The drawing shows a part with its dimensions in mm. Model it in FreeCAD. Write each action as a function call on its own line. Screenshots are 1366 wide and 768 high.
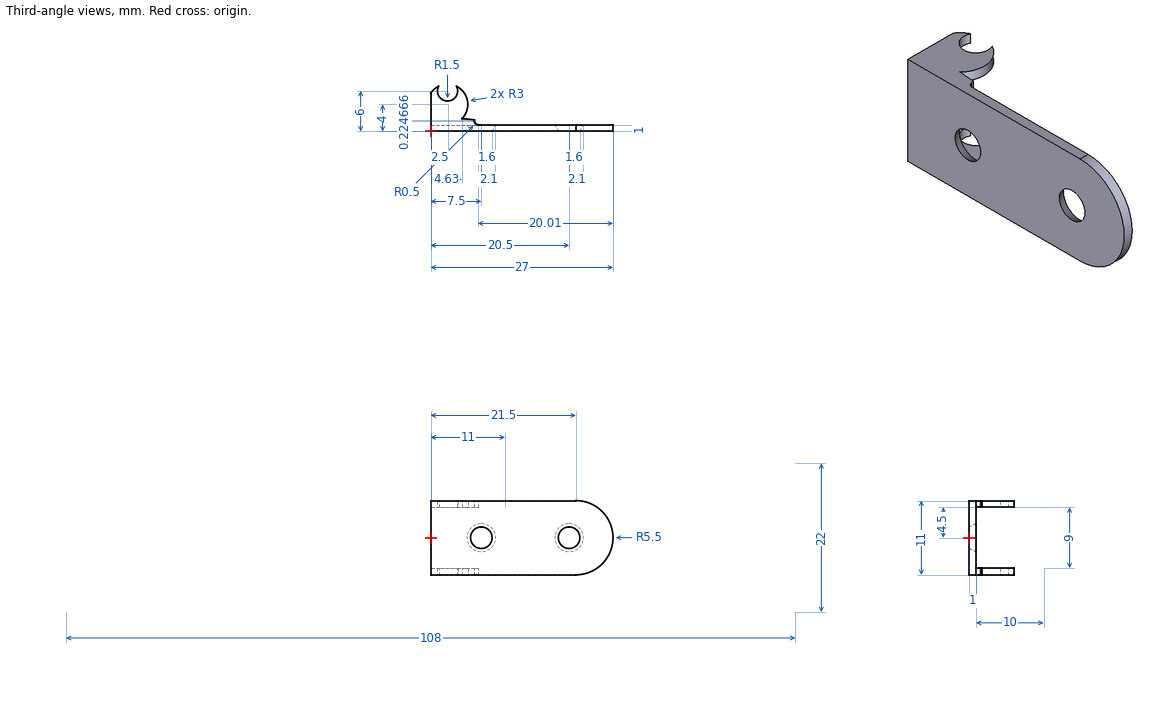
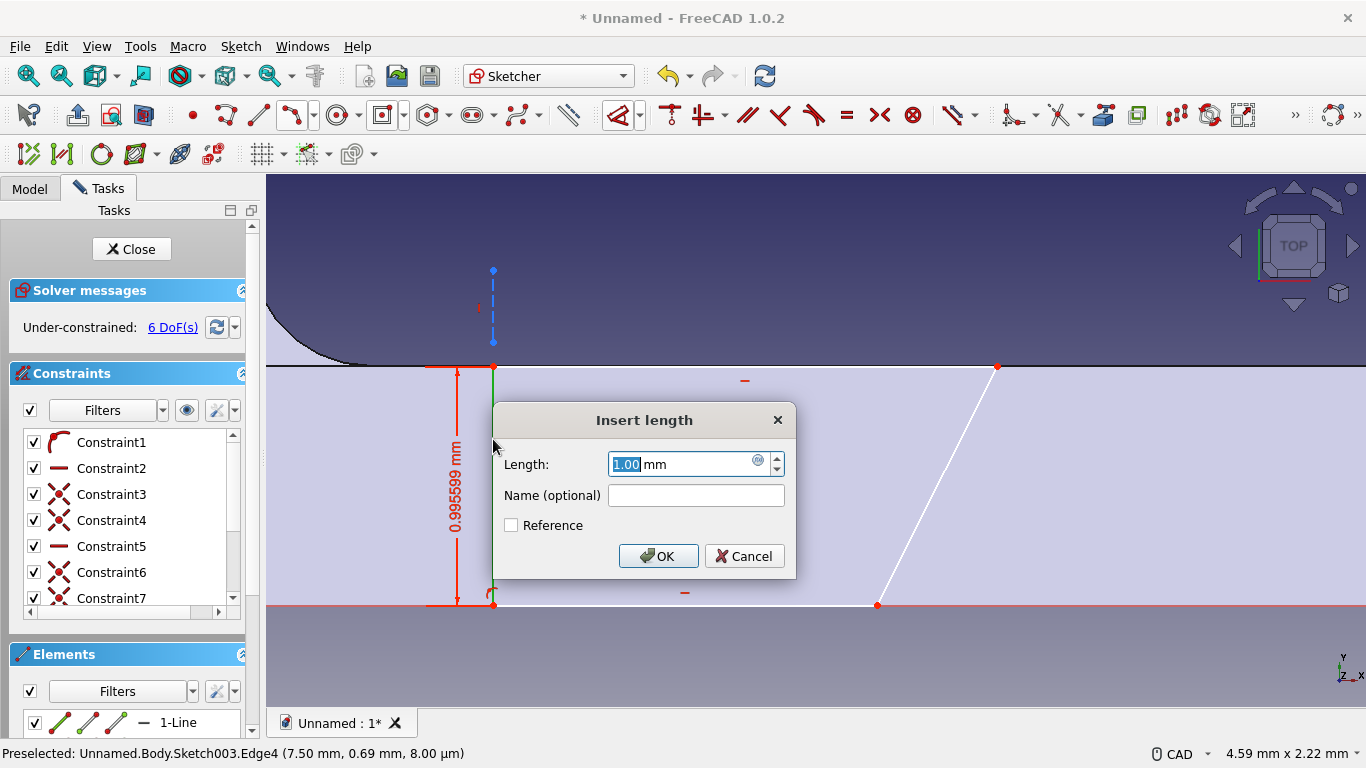
text(1)
key(Return)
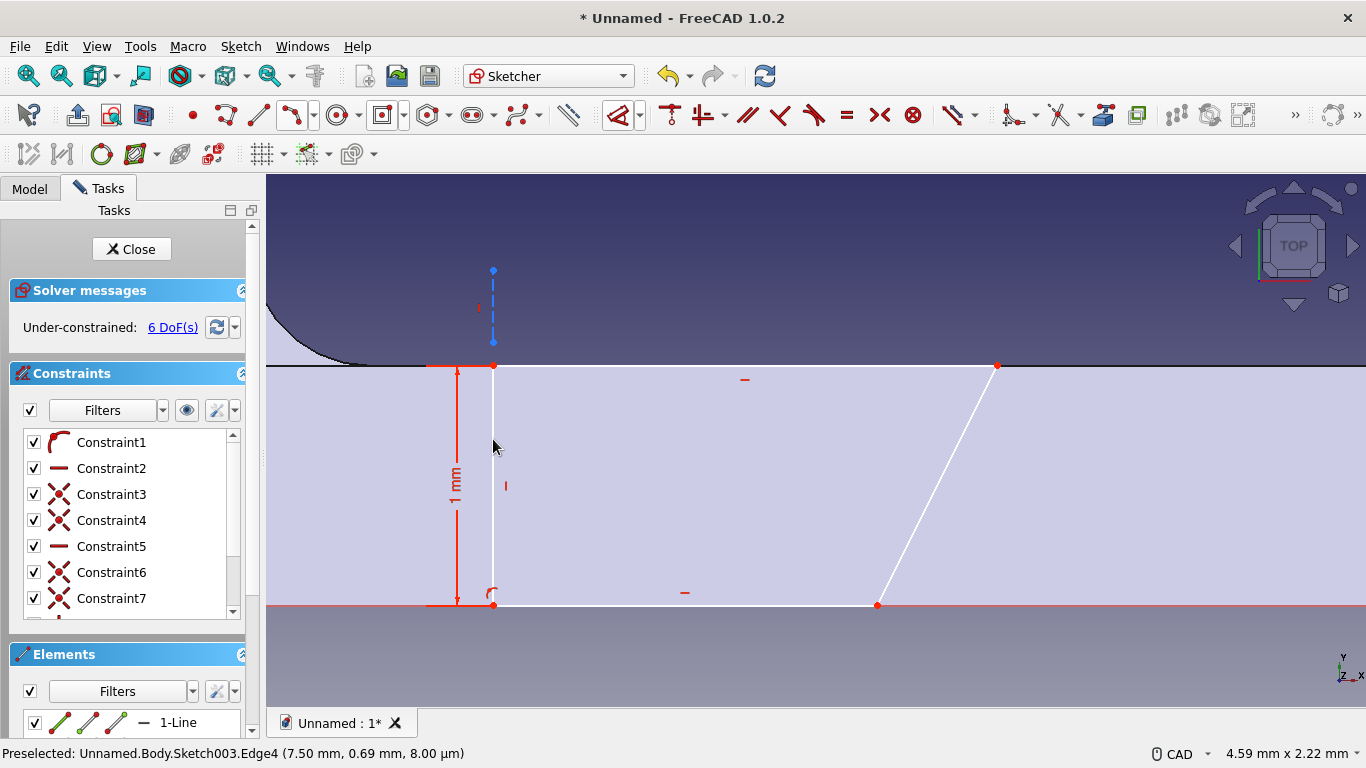
click(608, 606)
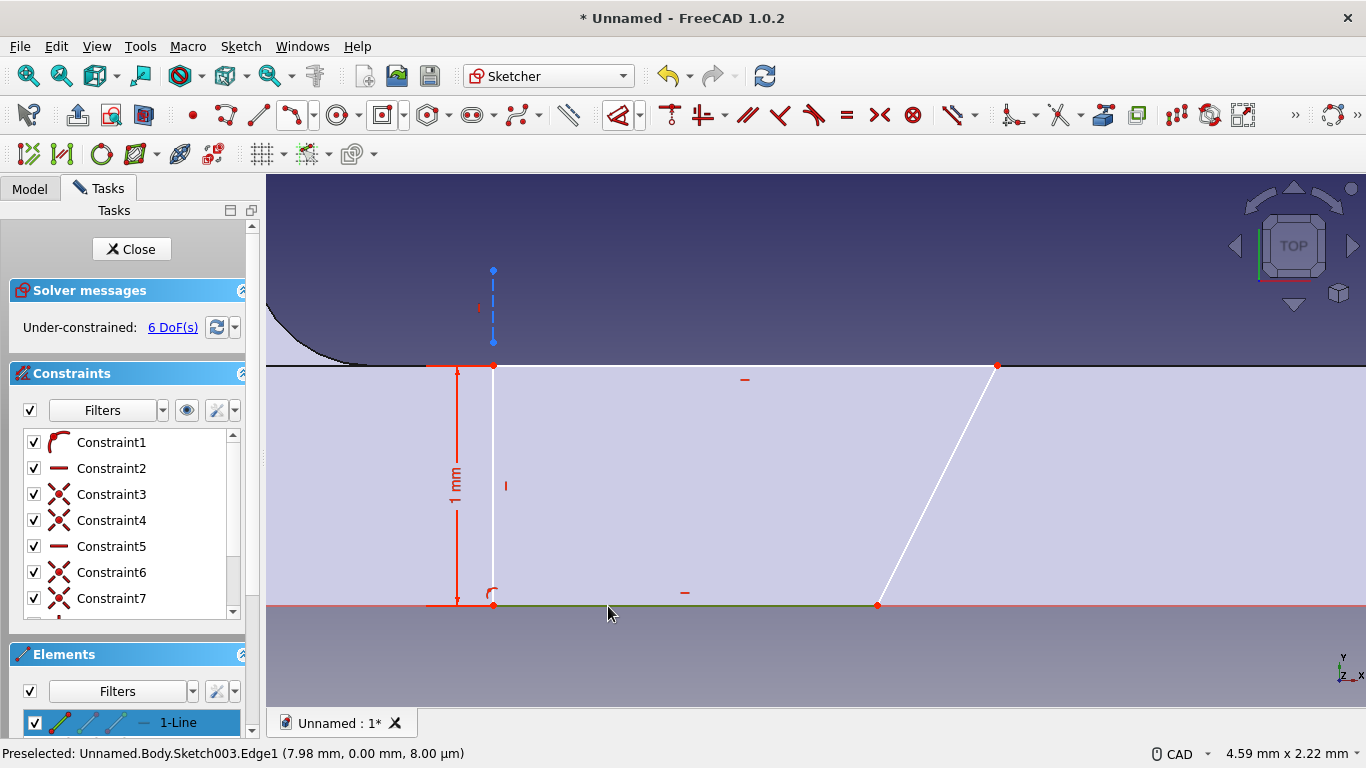
key(l)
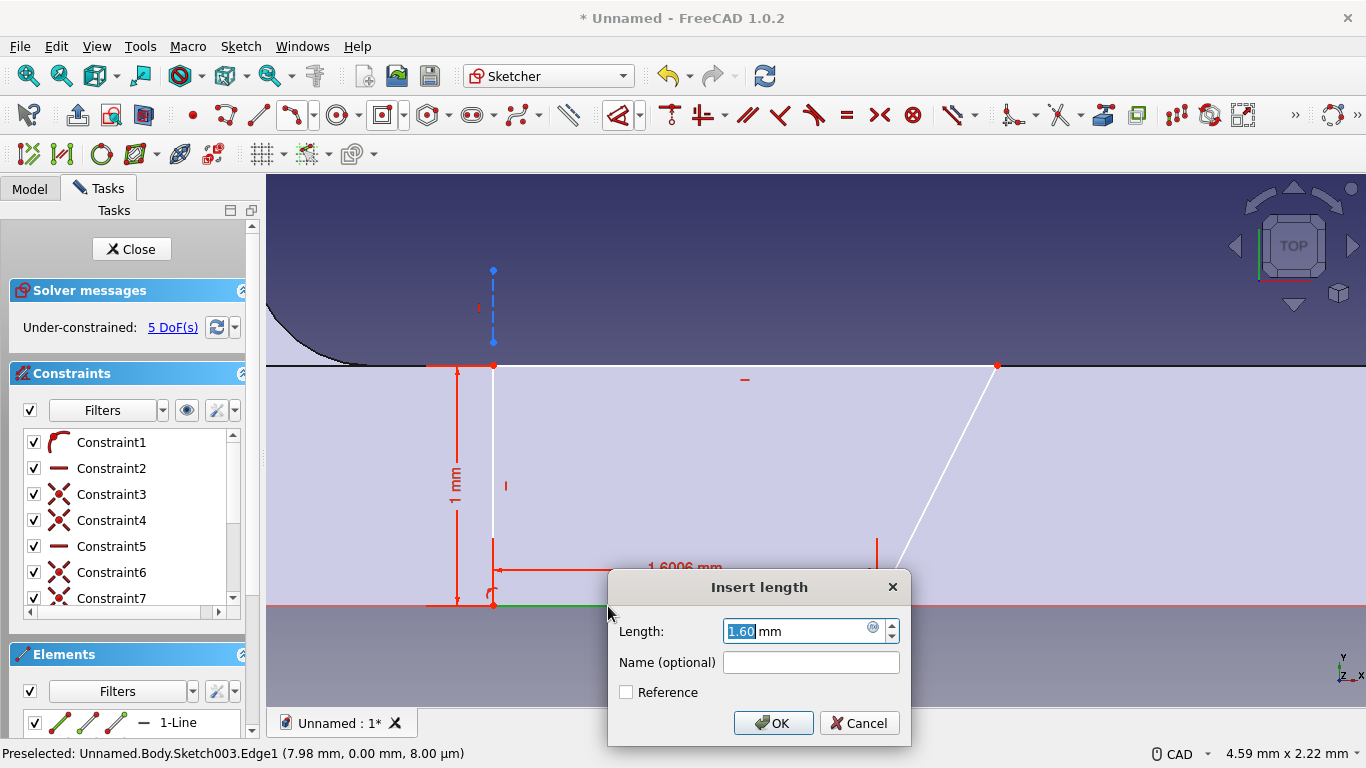
text(1.6)
key(Return)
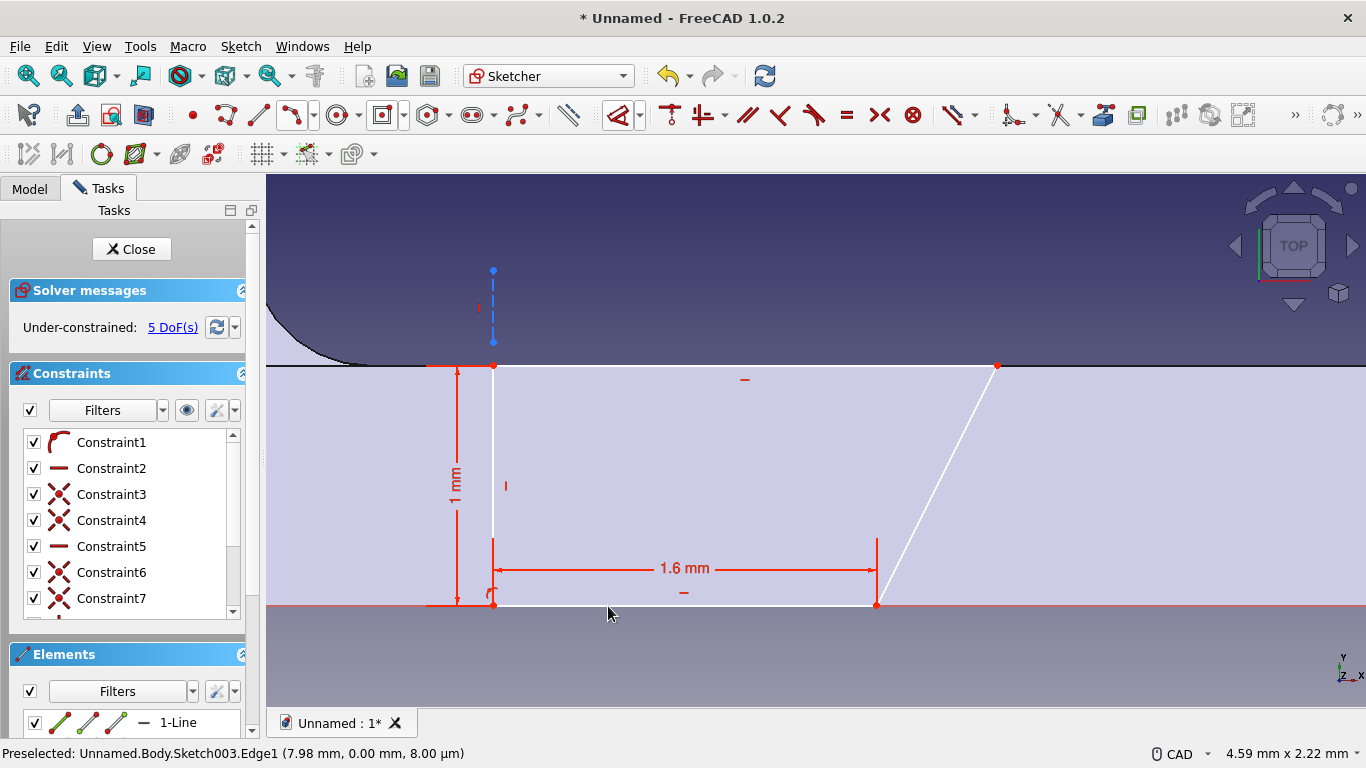
click(846, 366)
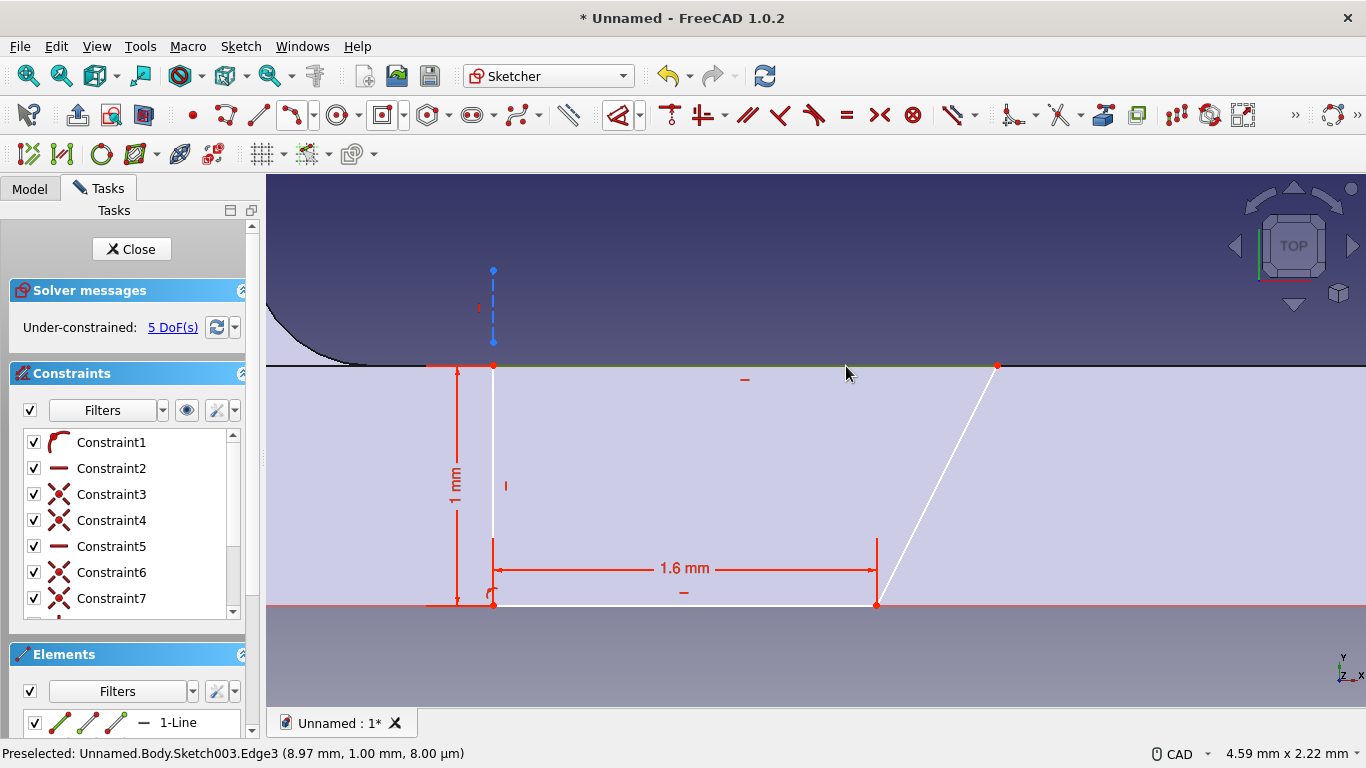
key(l)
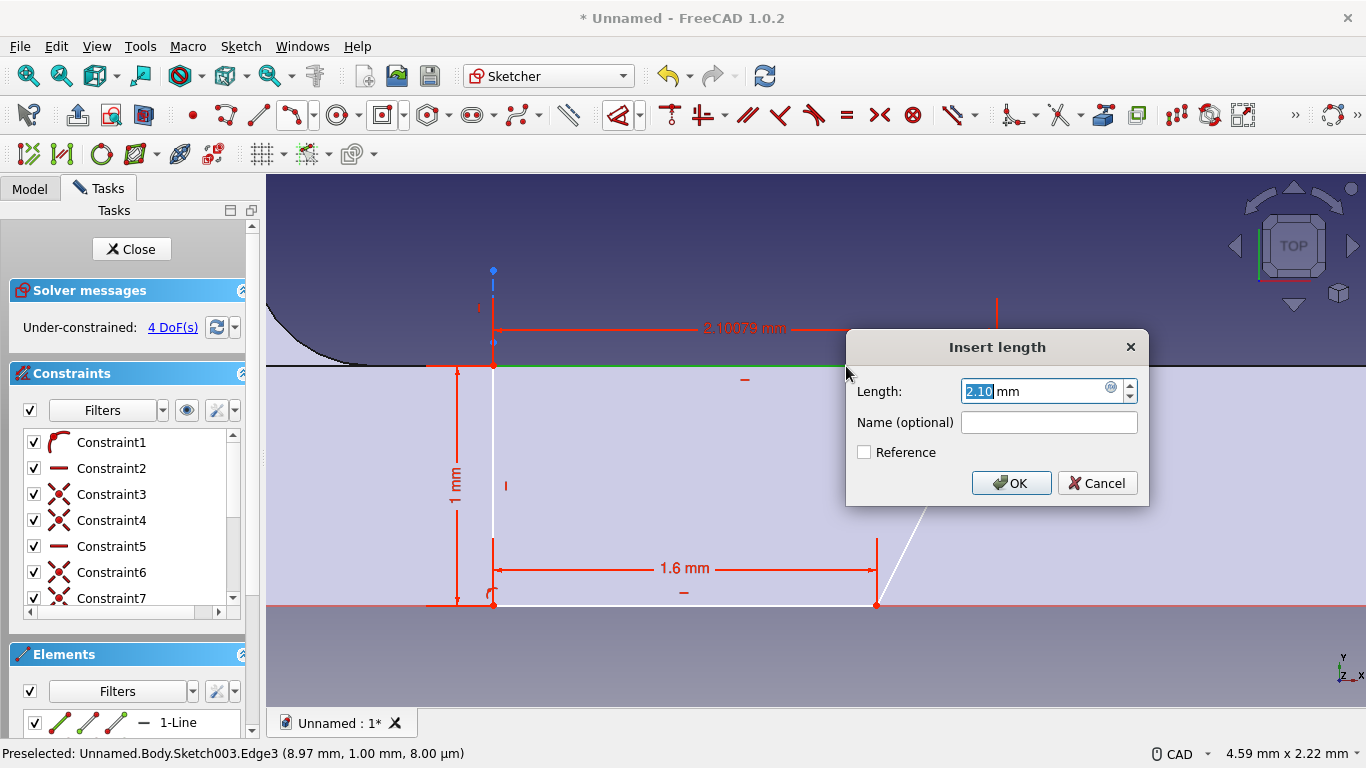
text(2.1)
key(Return)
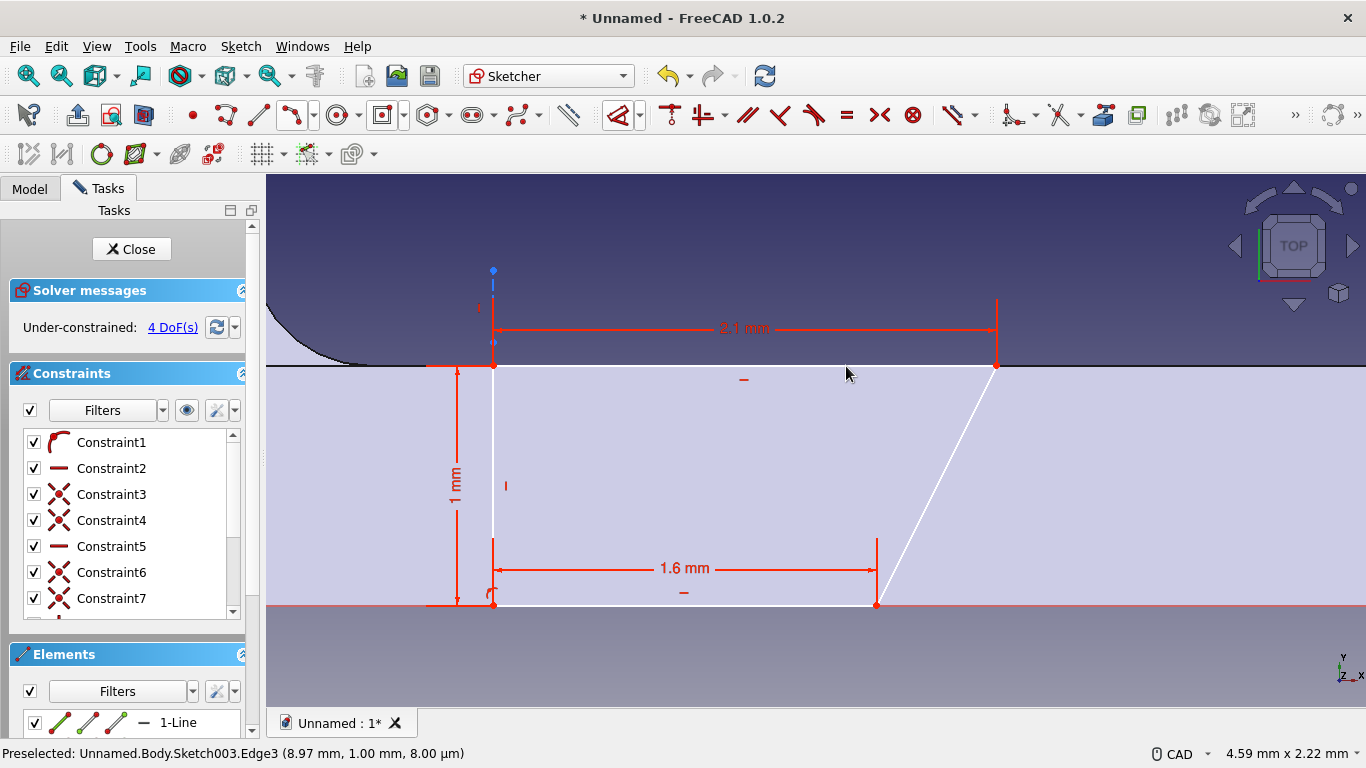
click(493, 606)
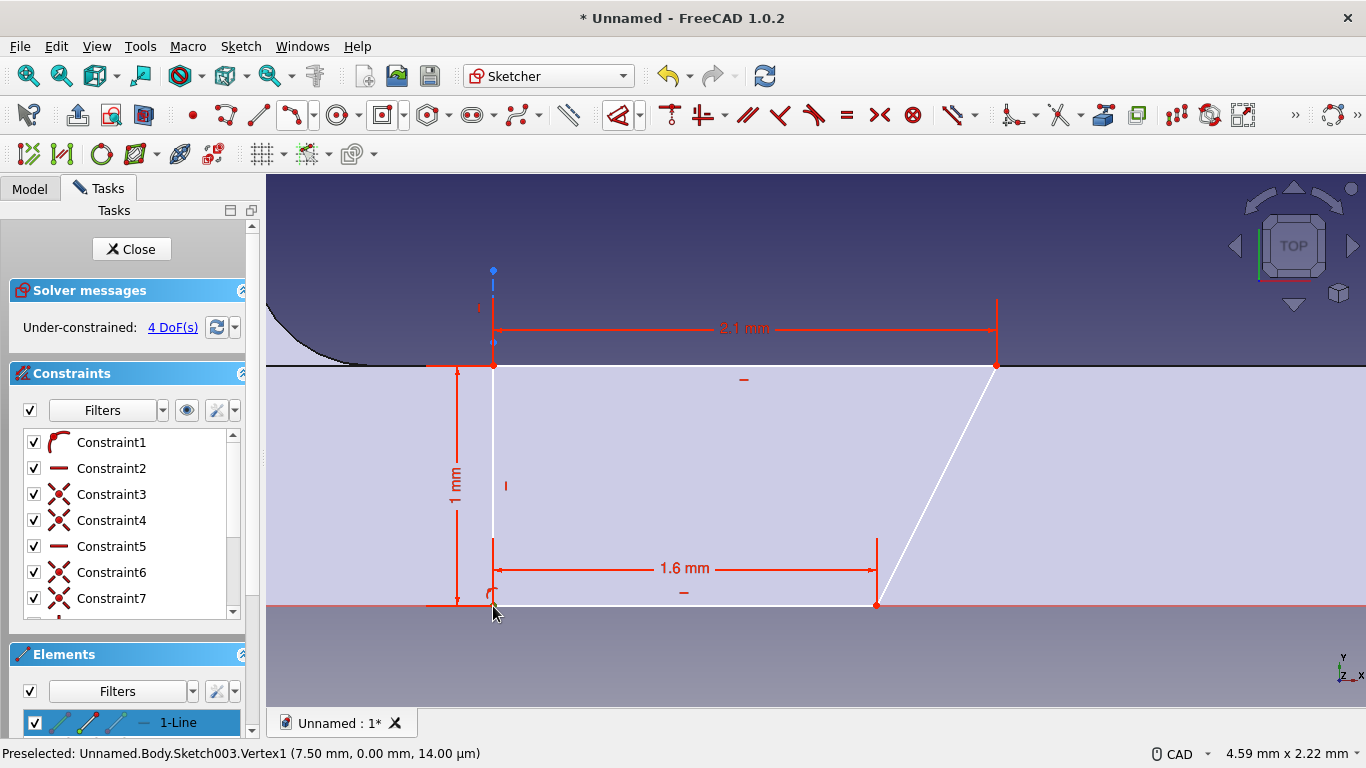
key(l)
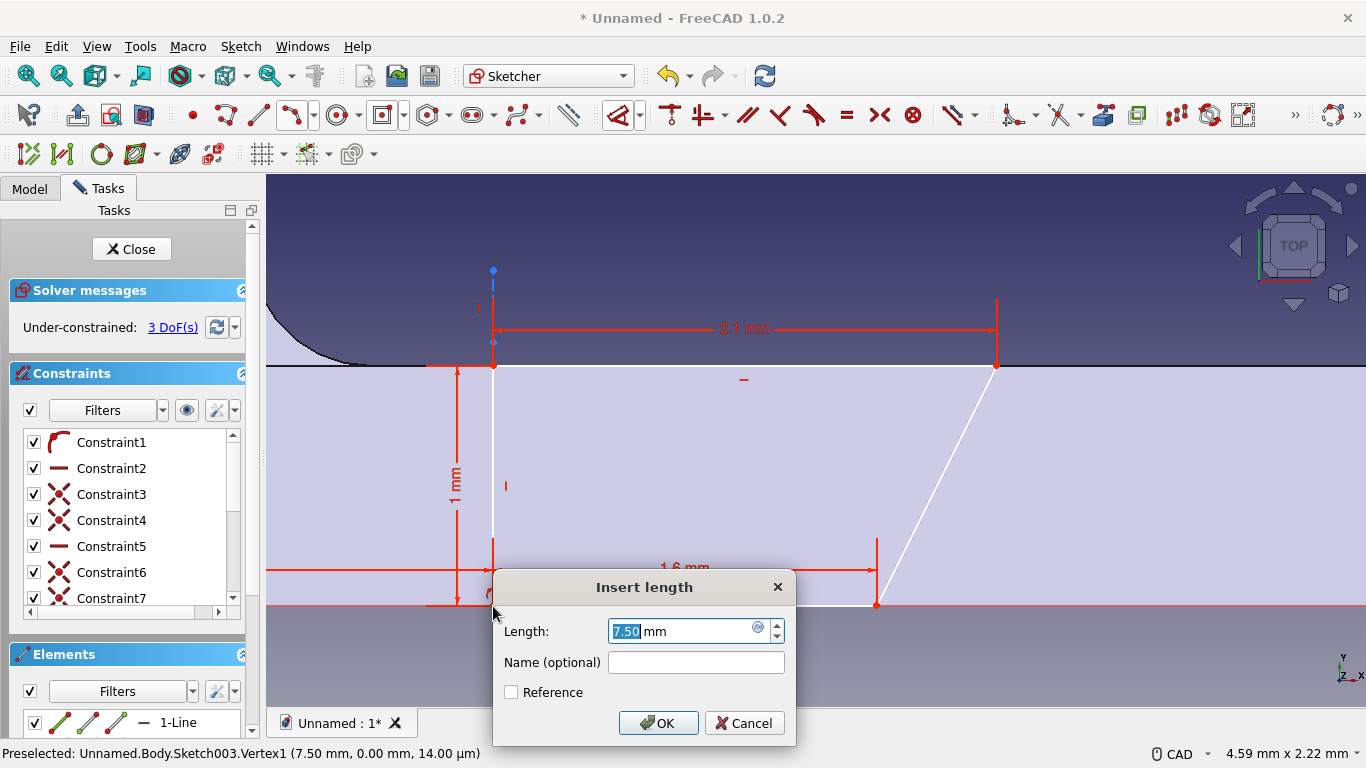
text(7.5)
key(Return)